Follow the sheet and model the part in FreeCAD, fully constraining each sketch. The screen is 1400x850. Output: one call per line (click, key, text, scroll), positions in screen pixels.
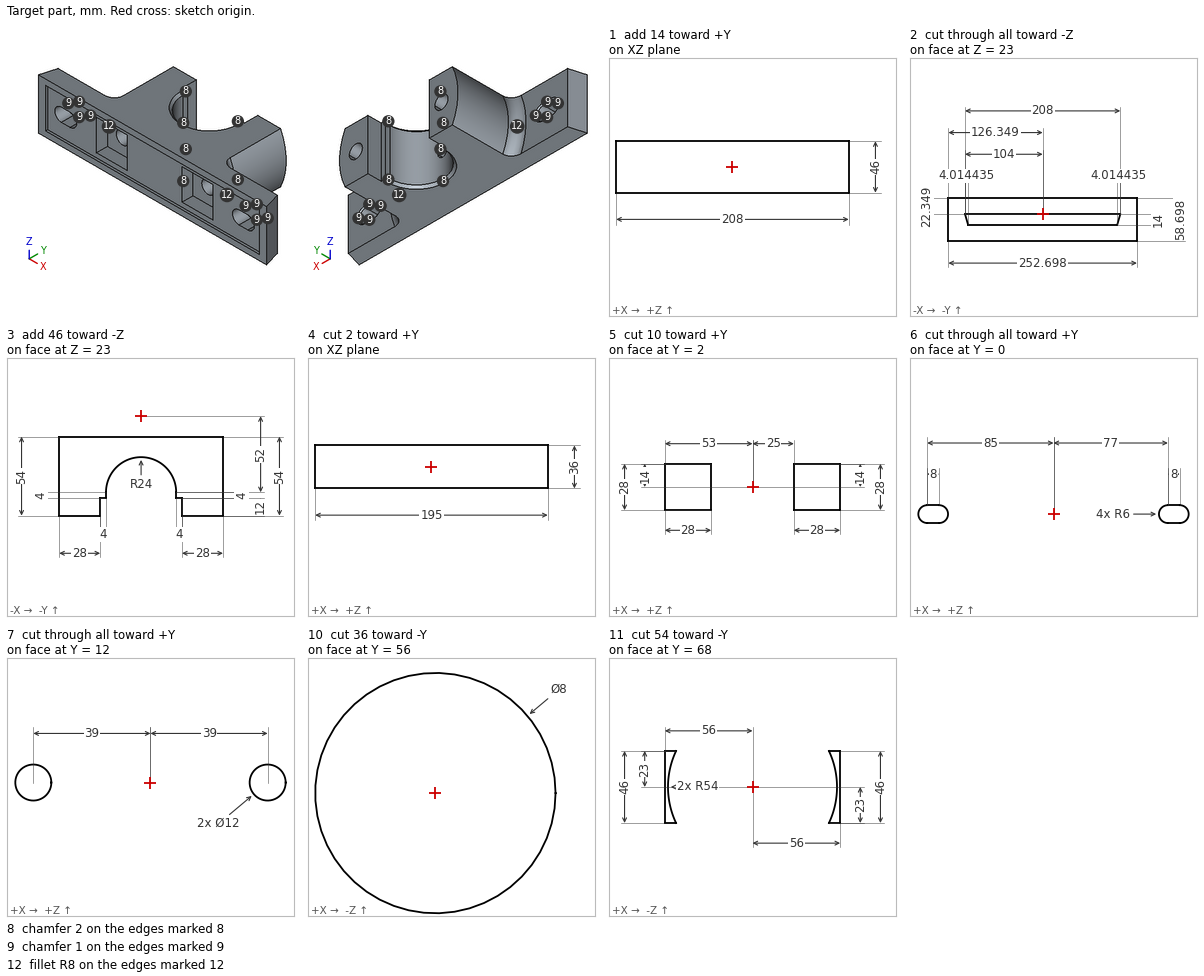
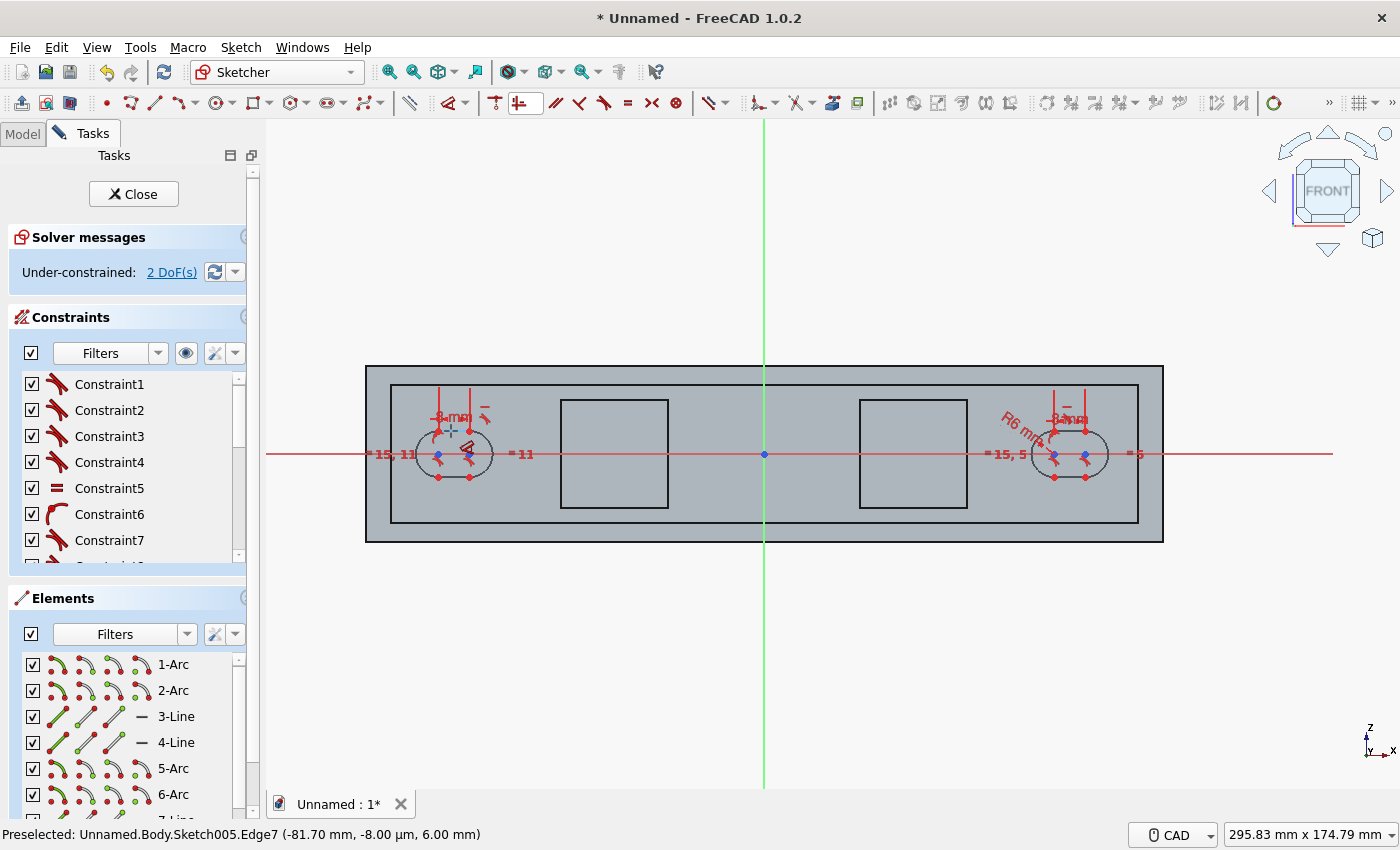
click(1054, 431)
click(909, 397)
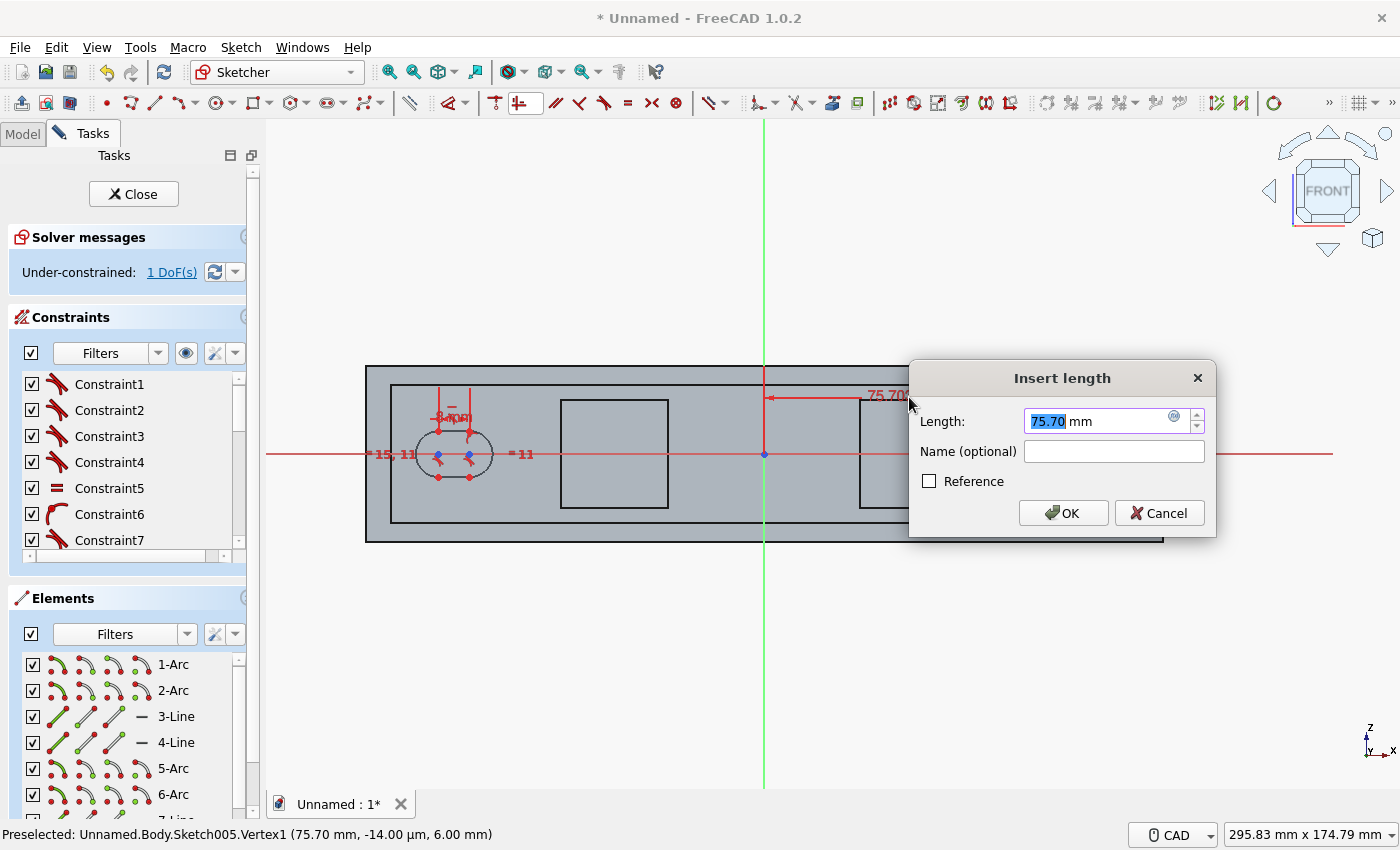
text(77)
key(Return)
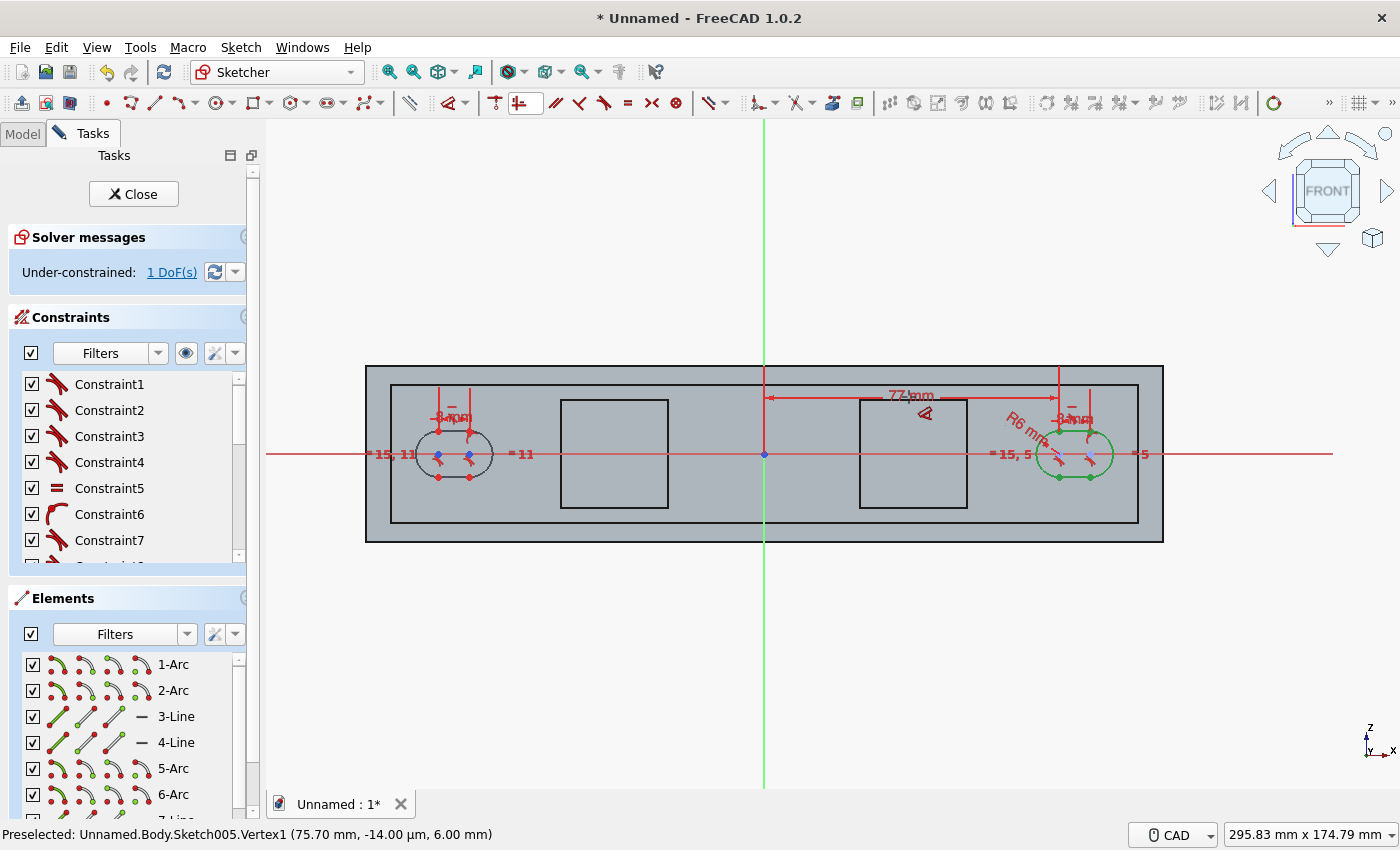
click(439, 431)
click(602, 397)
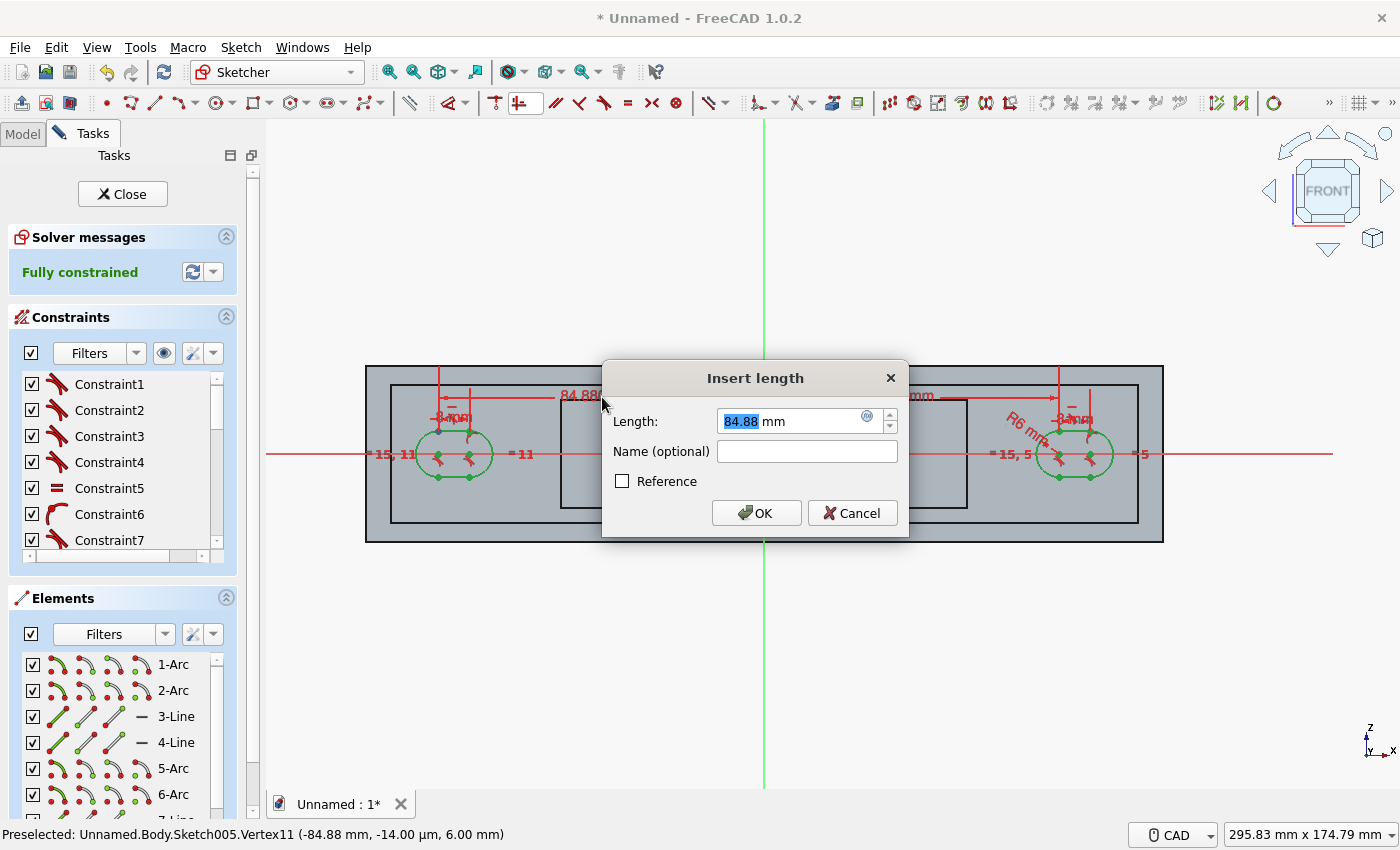
text(85)
key(Return)
key(Escape)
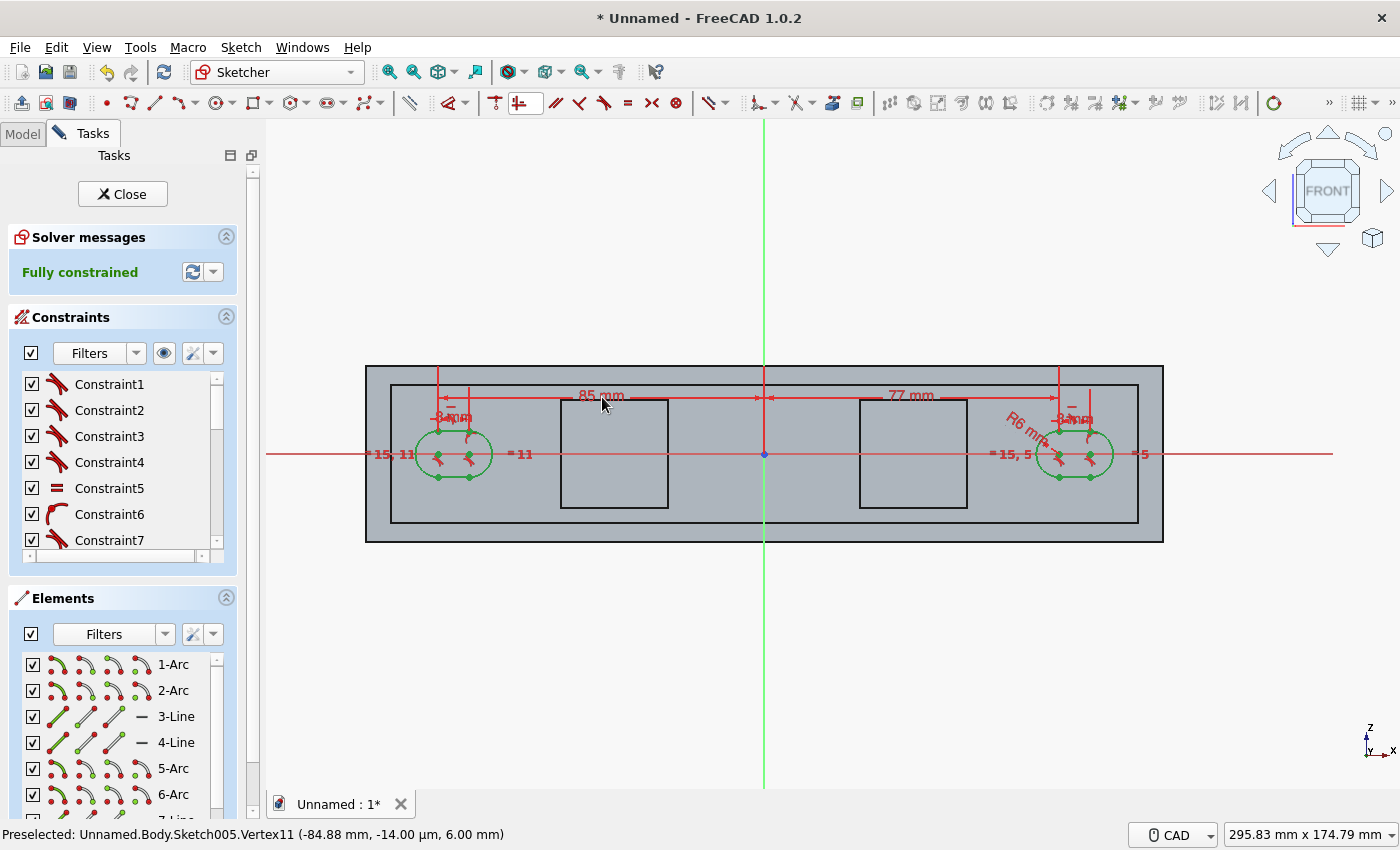
click(123, 194)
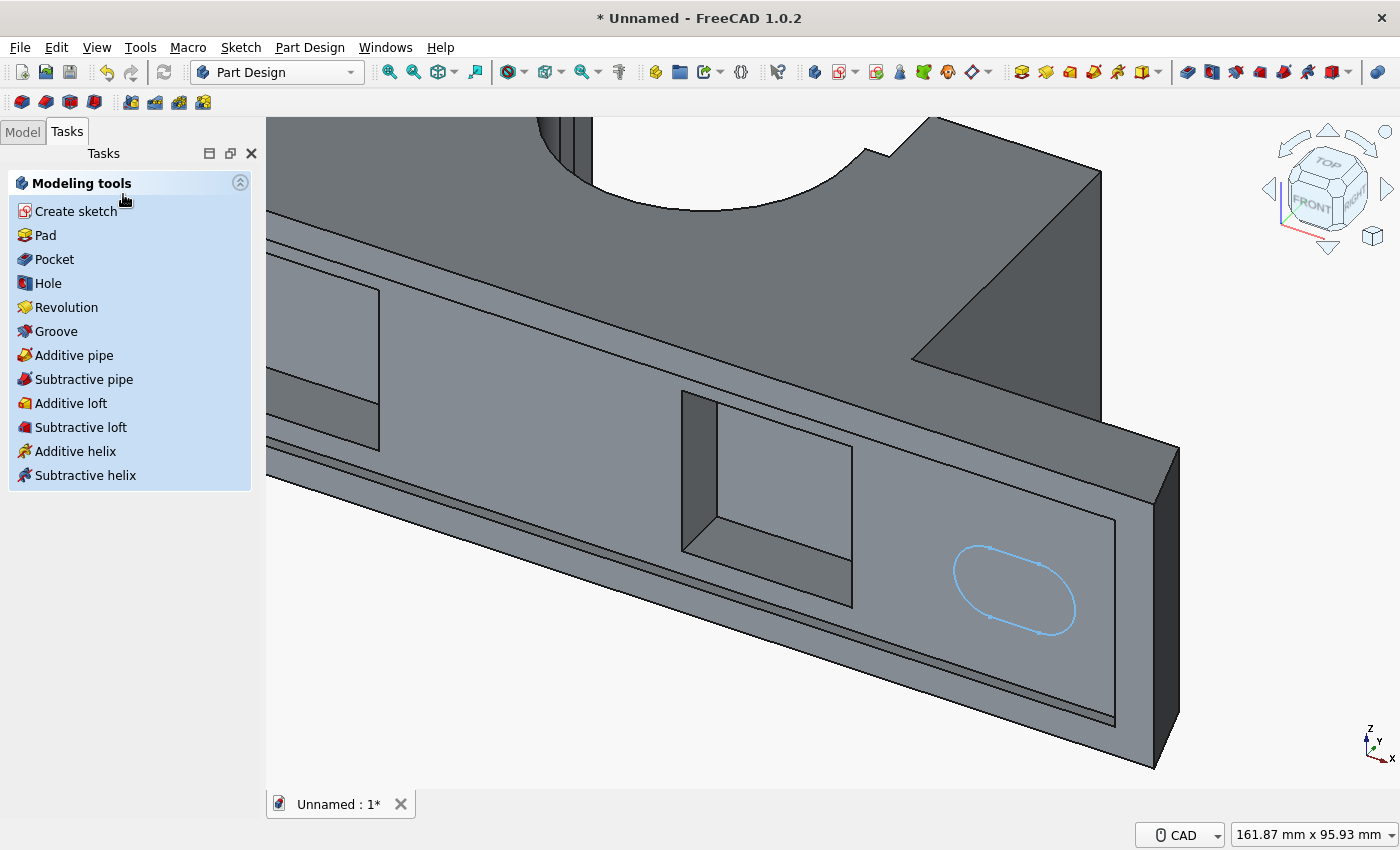
click(1188, 72)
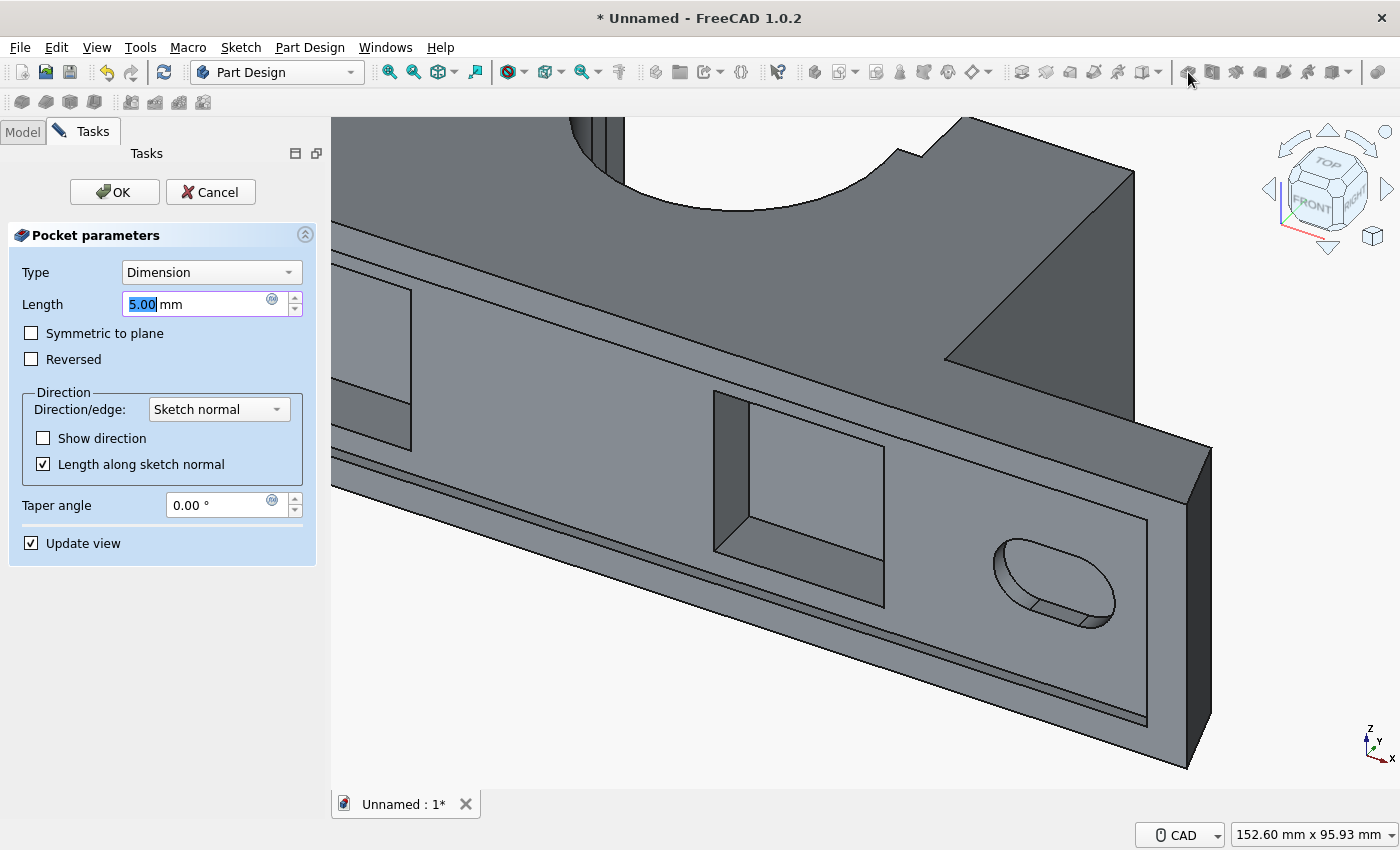
click(212, 272)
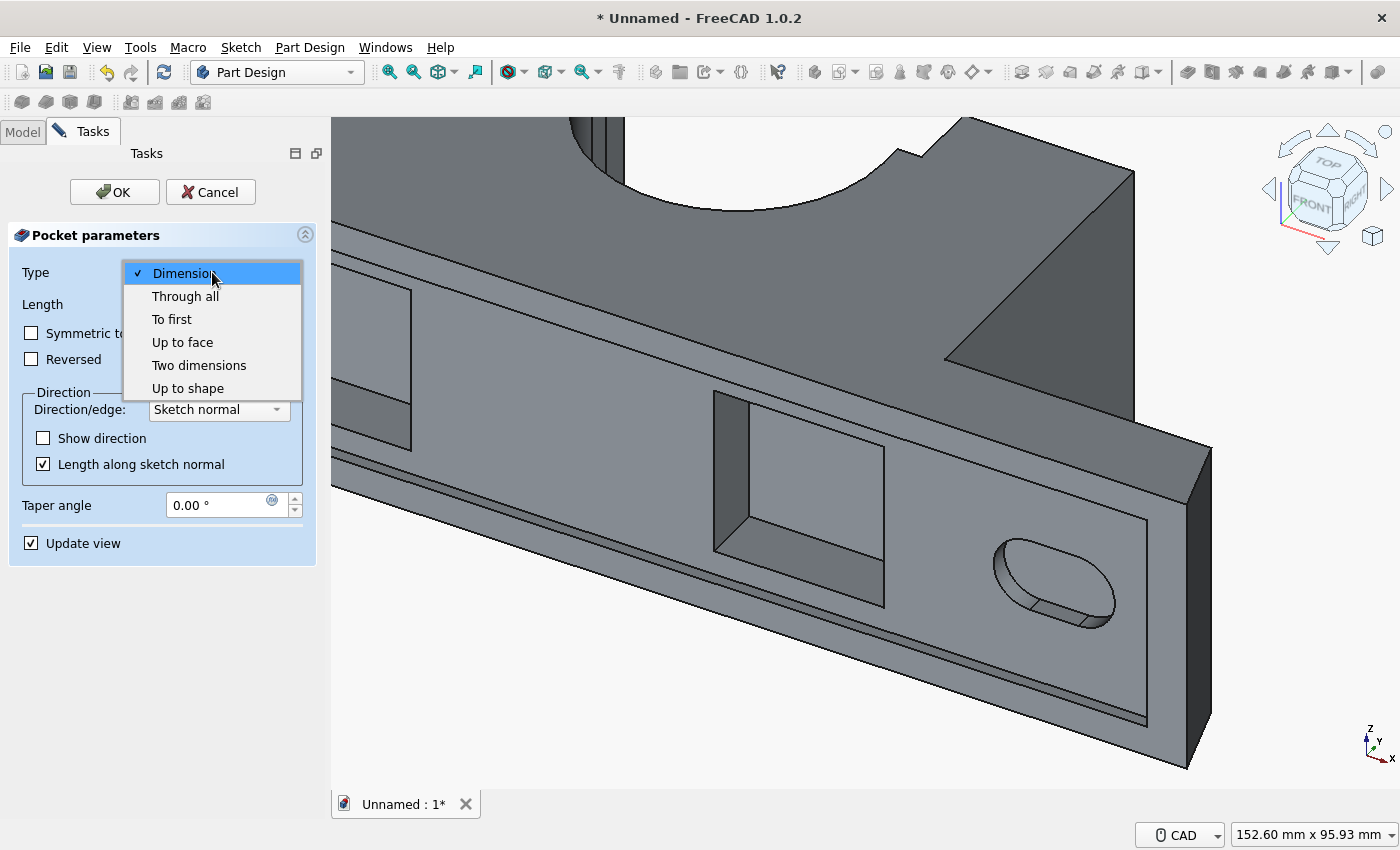
click(212, 296)